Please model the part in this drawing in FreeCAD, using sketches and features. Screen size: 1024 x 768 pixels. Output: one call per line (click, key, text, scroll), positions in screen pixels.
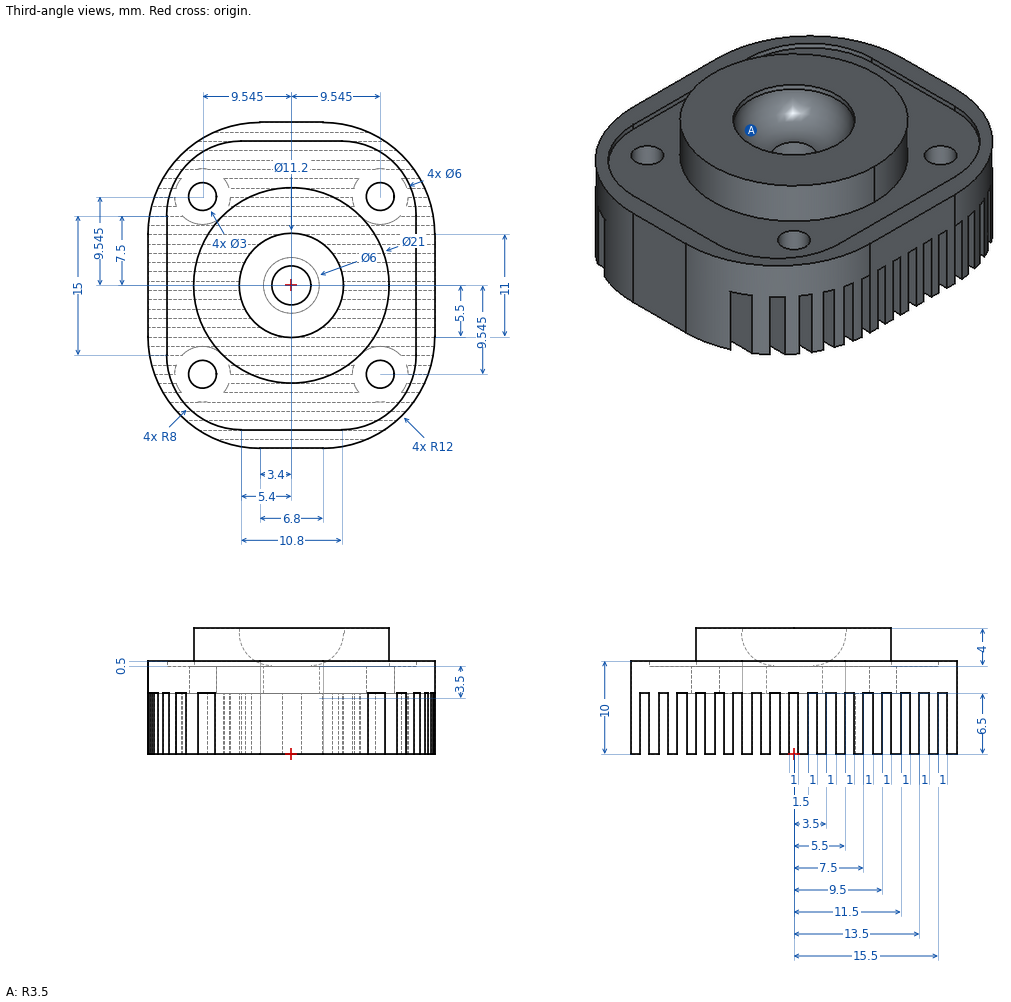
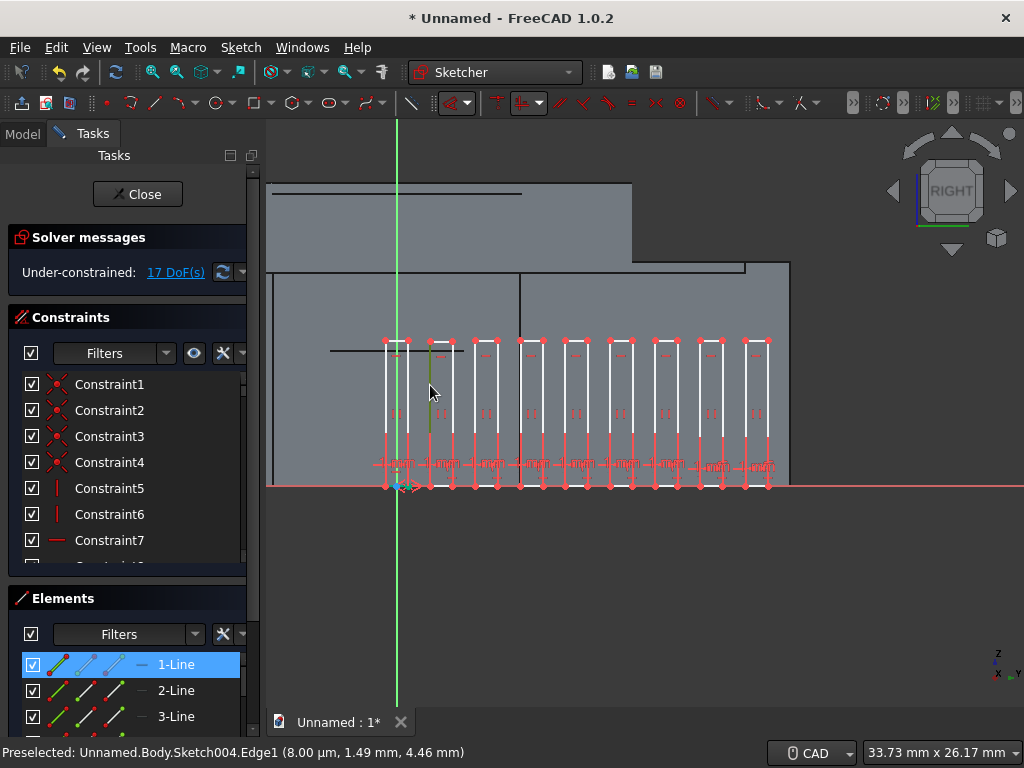
key(i)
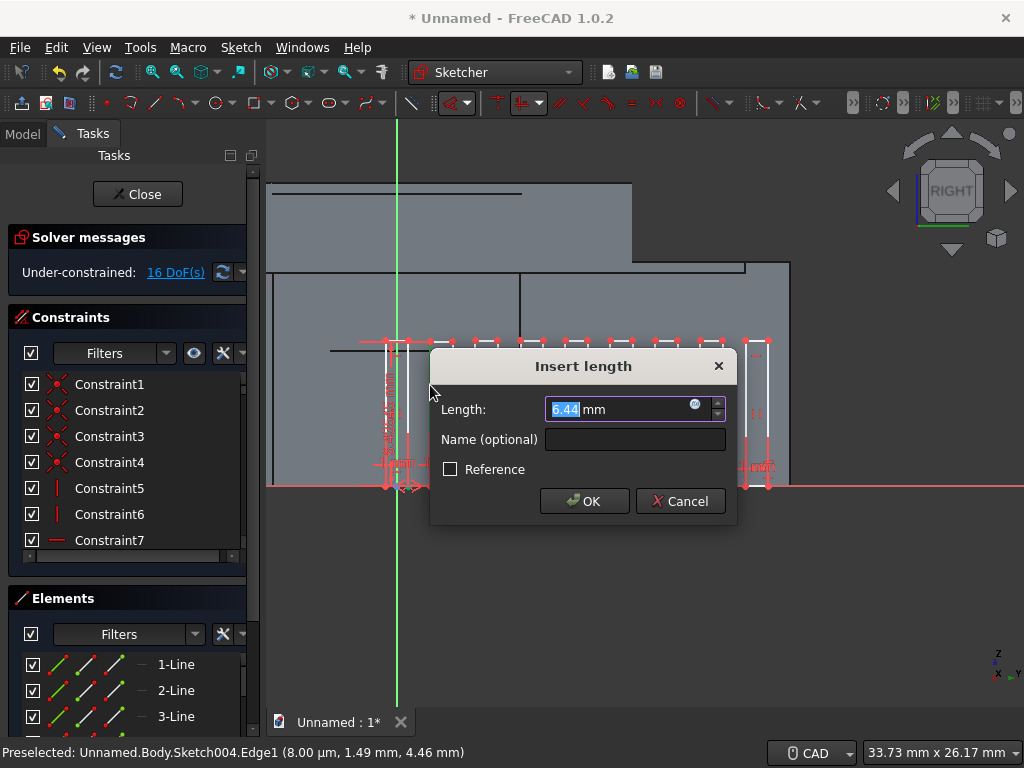
text(6.5)
key(Return)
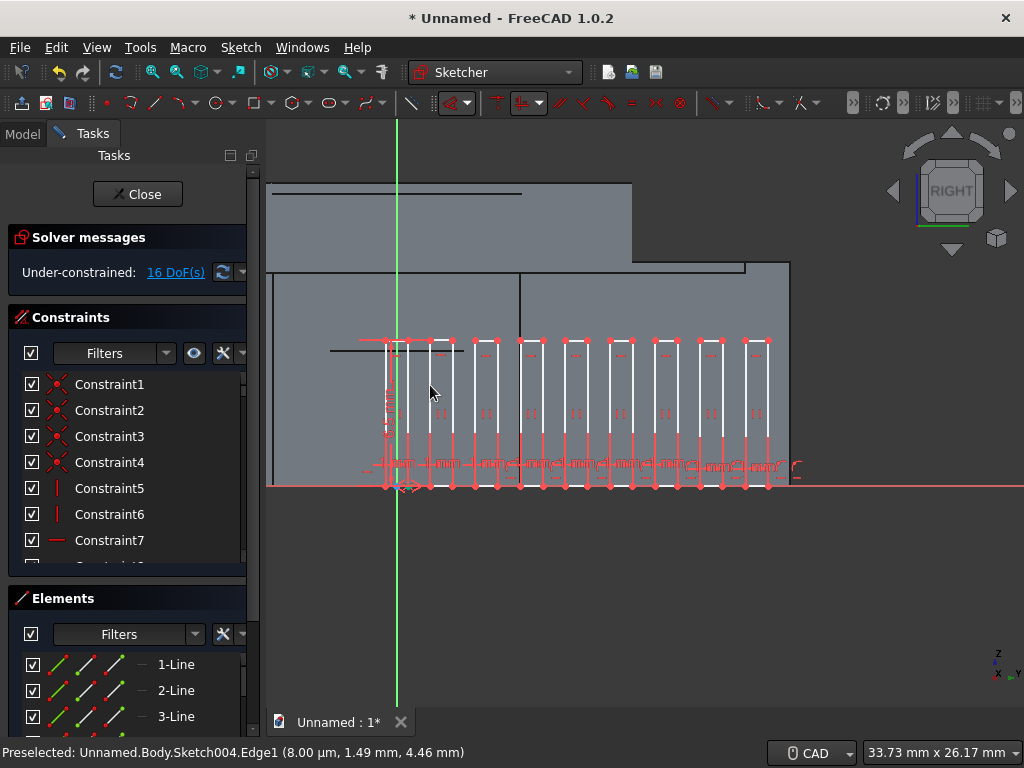
scroll(386, 384, up, 2)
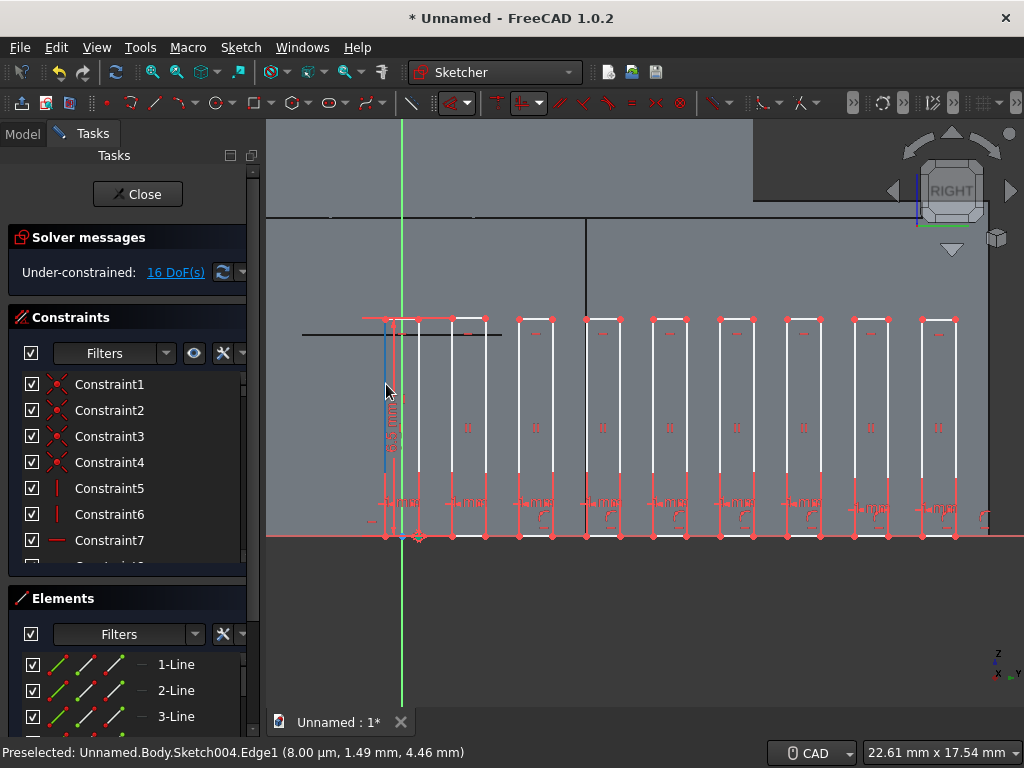
click(385, 384)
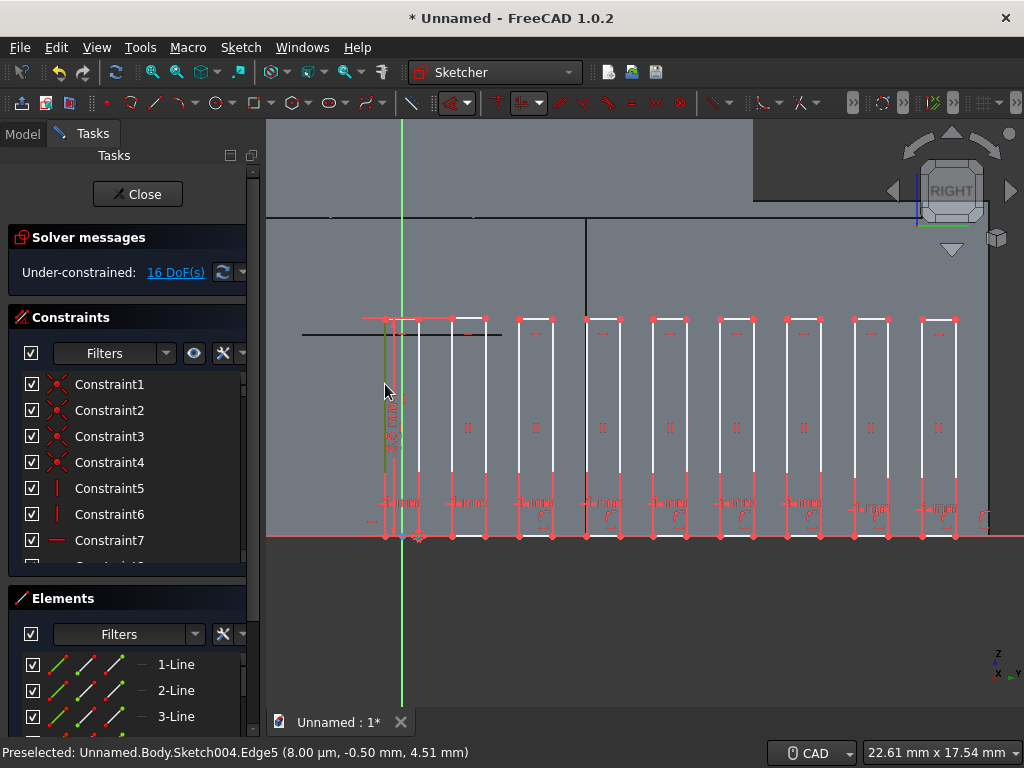
key(i)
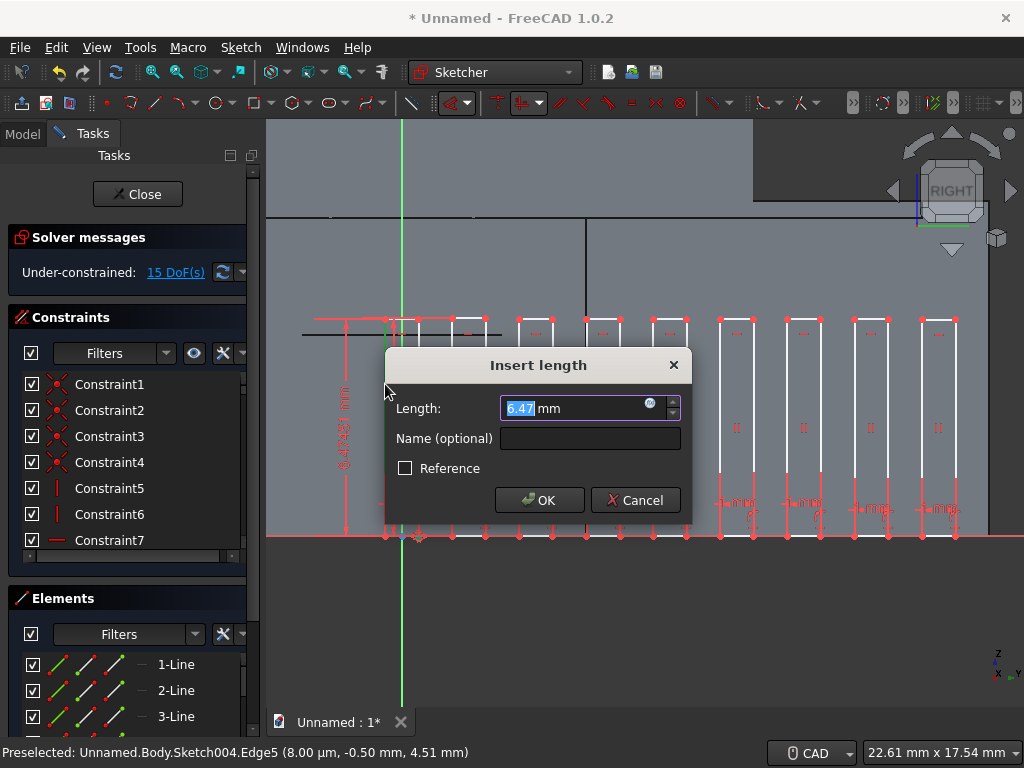
text(6.5)
key(Return)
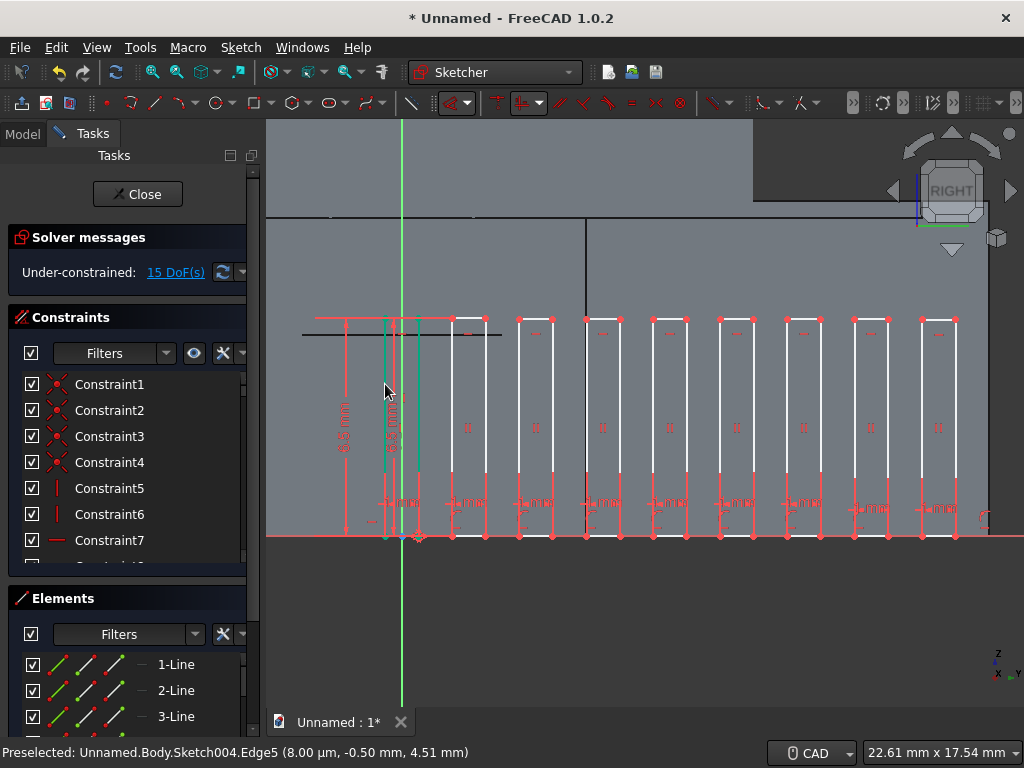
click(519, 384)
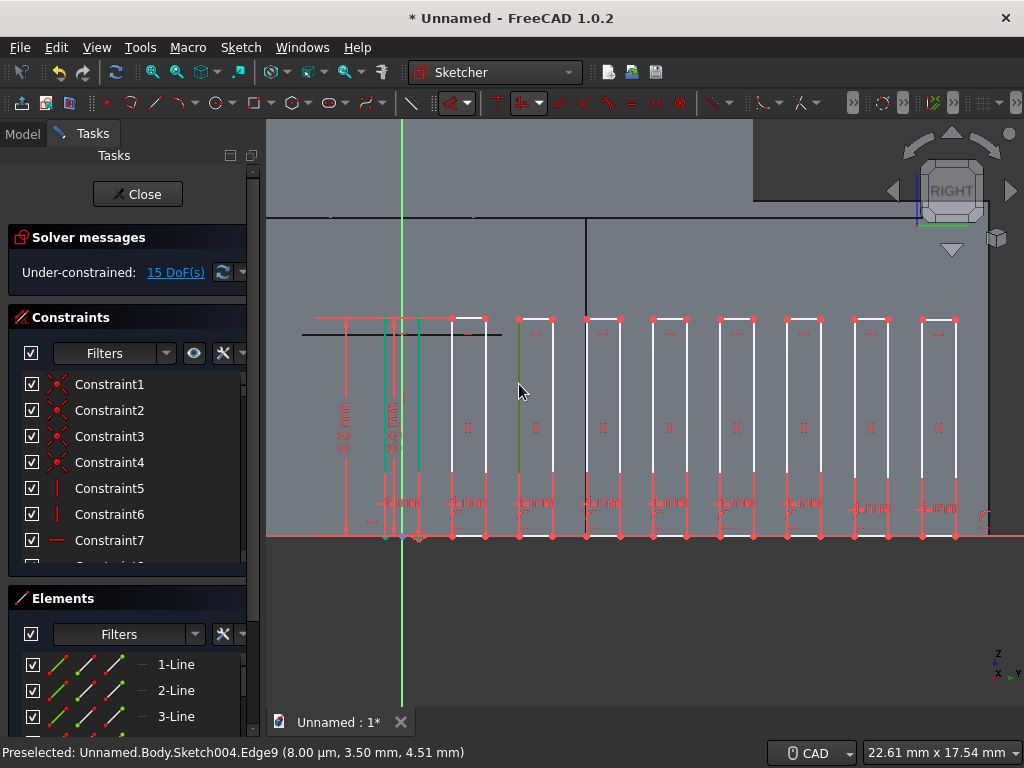
click(470, 104)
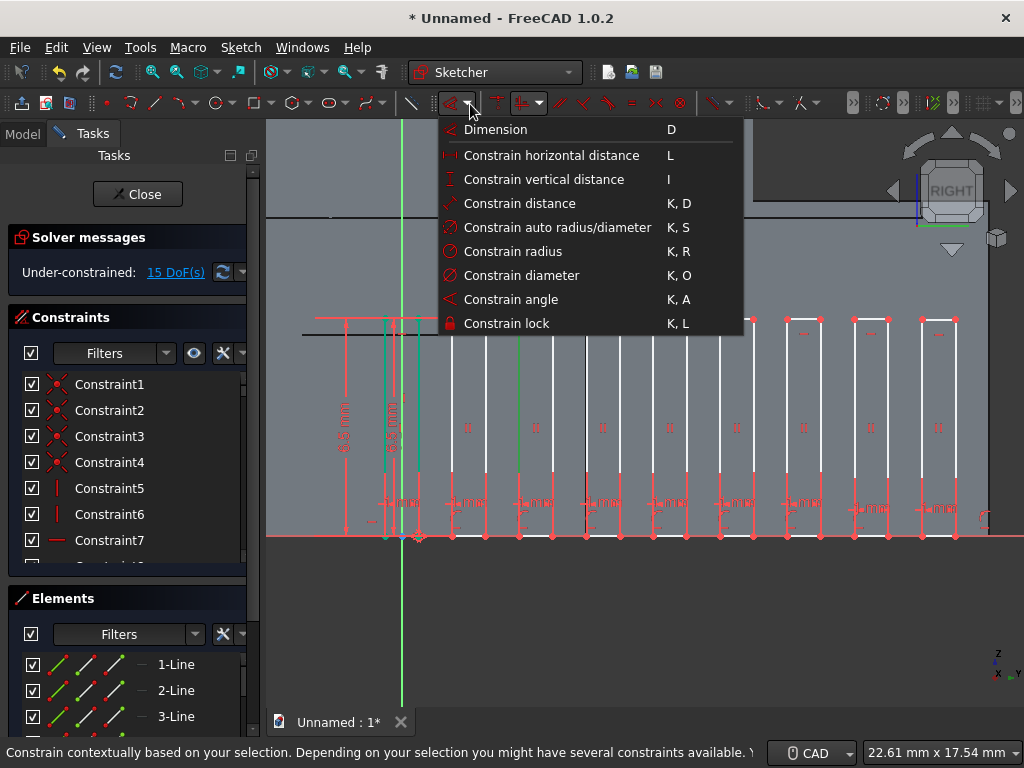
click(591, 179)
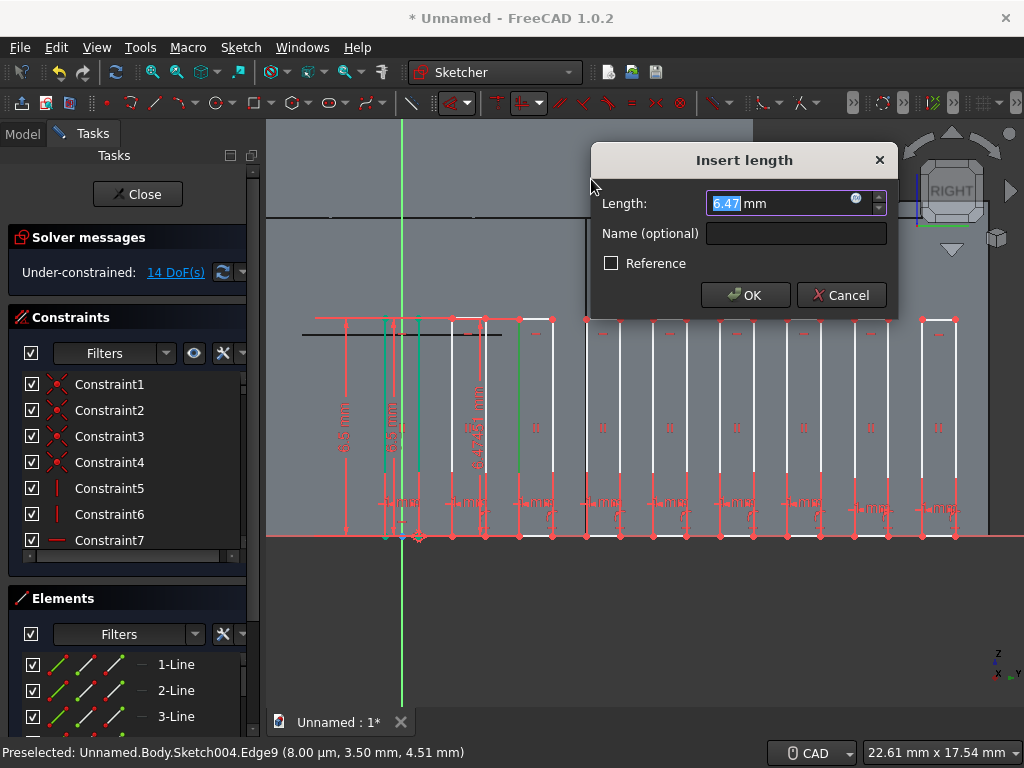
text(6.5)
key(Return)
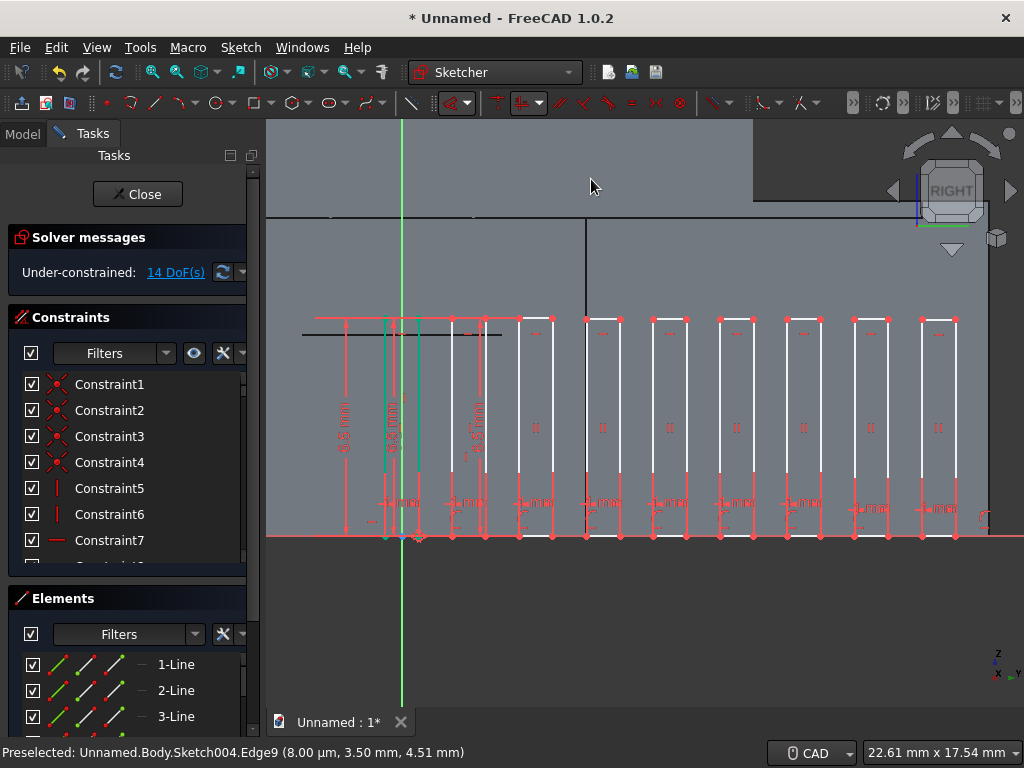
click(587, 384)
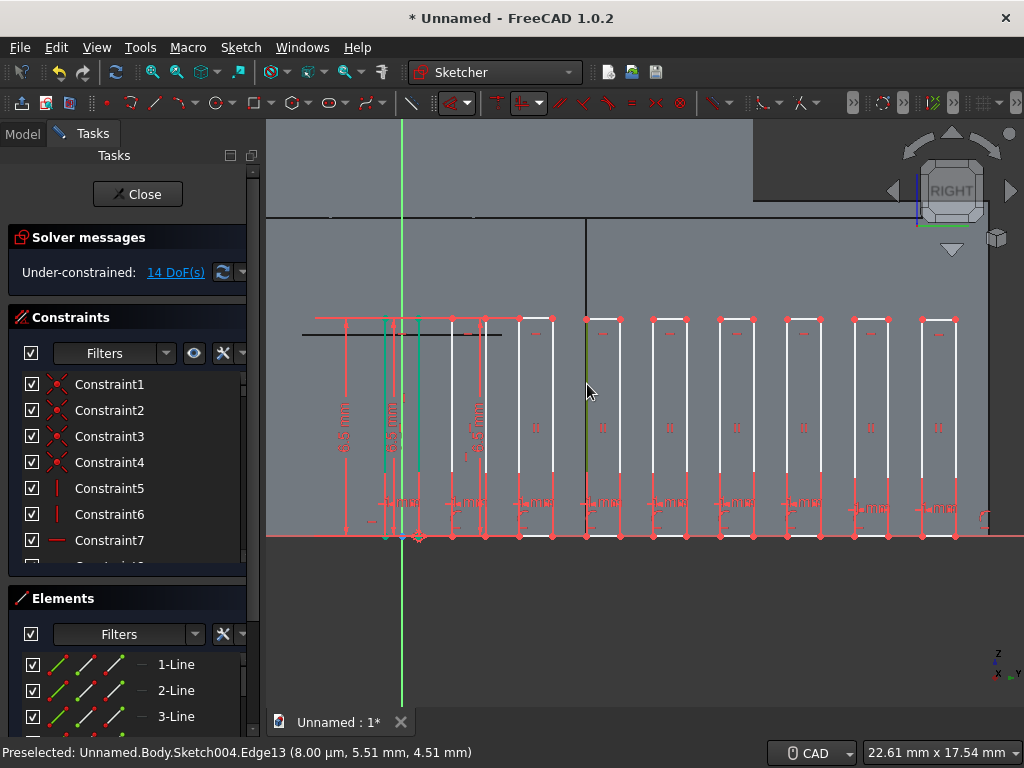
click(470, 104)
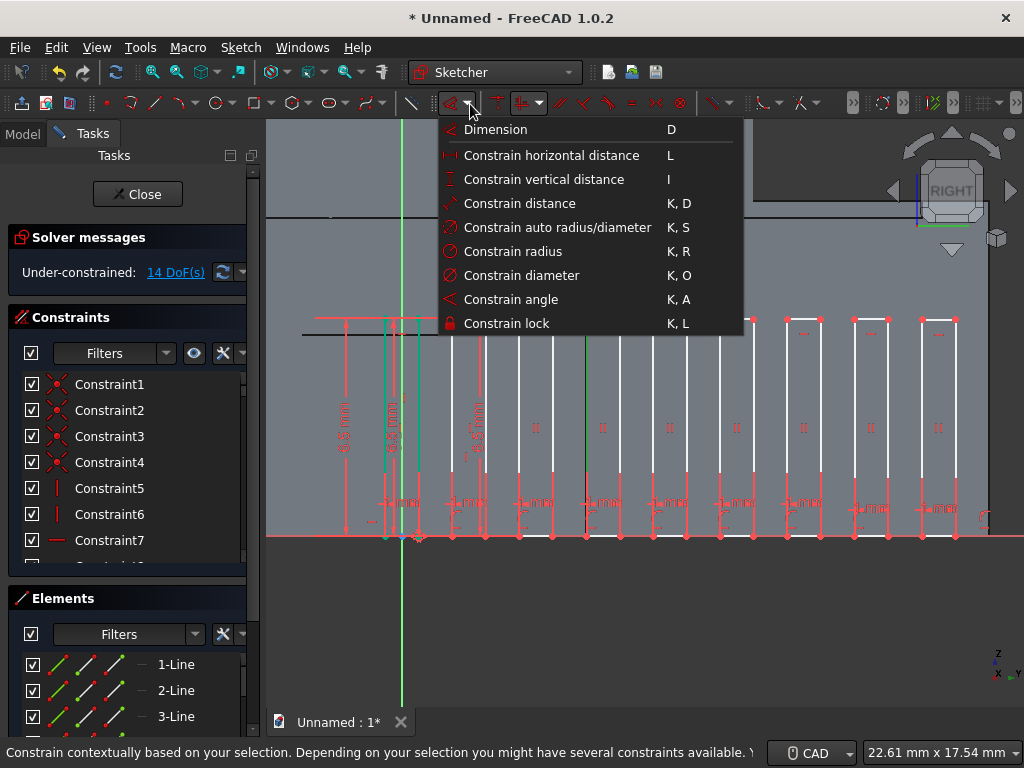
click(591, 179)